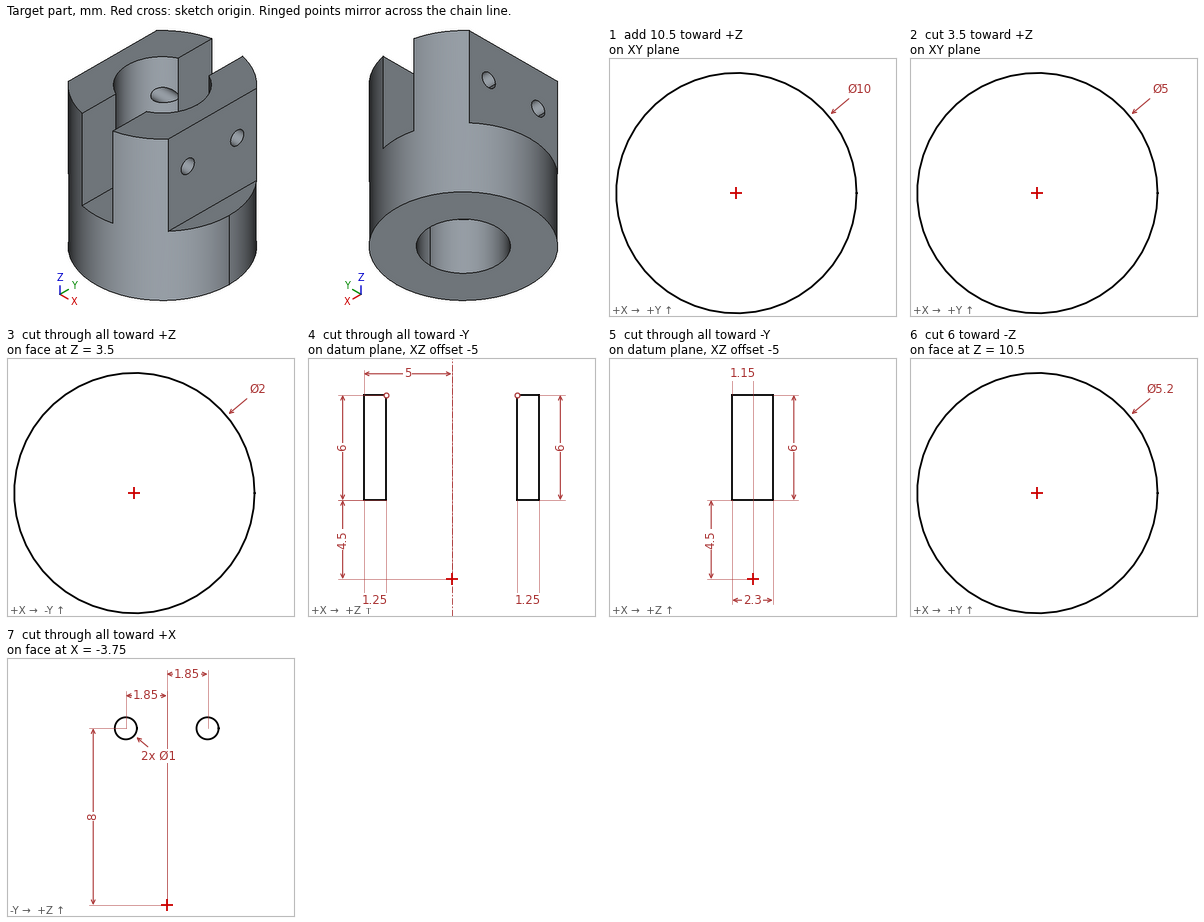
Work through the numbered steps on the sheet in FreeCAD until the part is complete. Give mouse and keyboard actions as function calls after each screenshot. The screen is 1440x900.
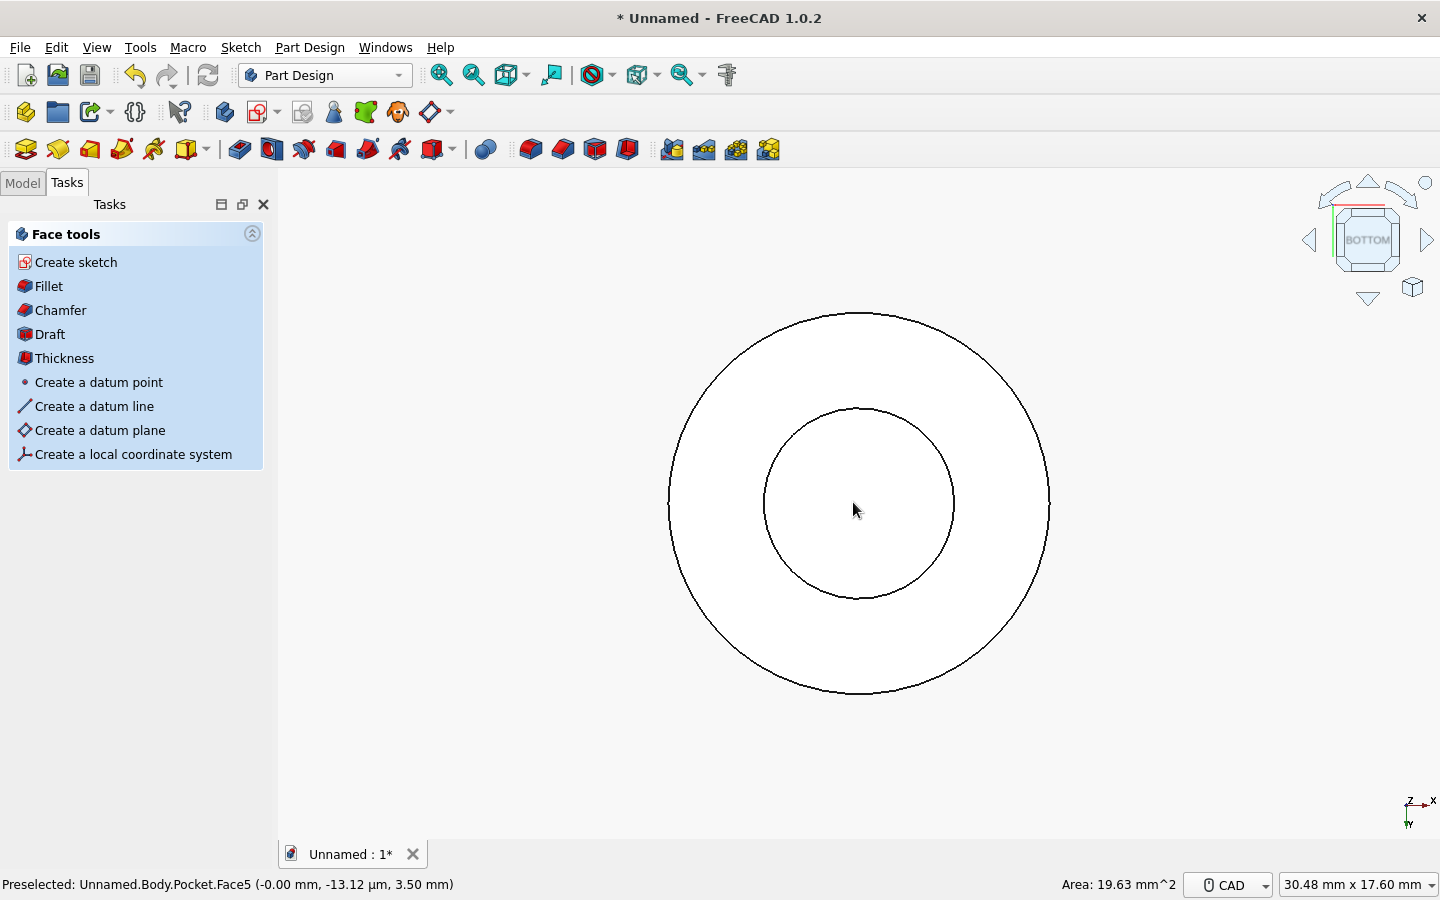
click(258, 112)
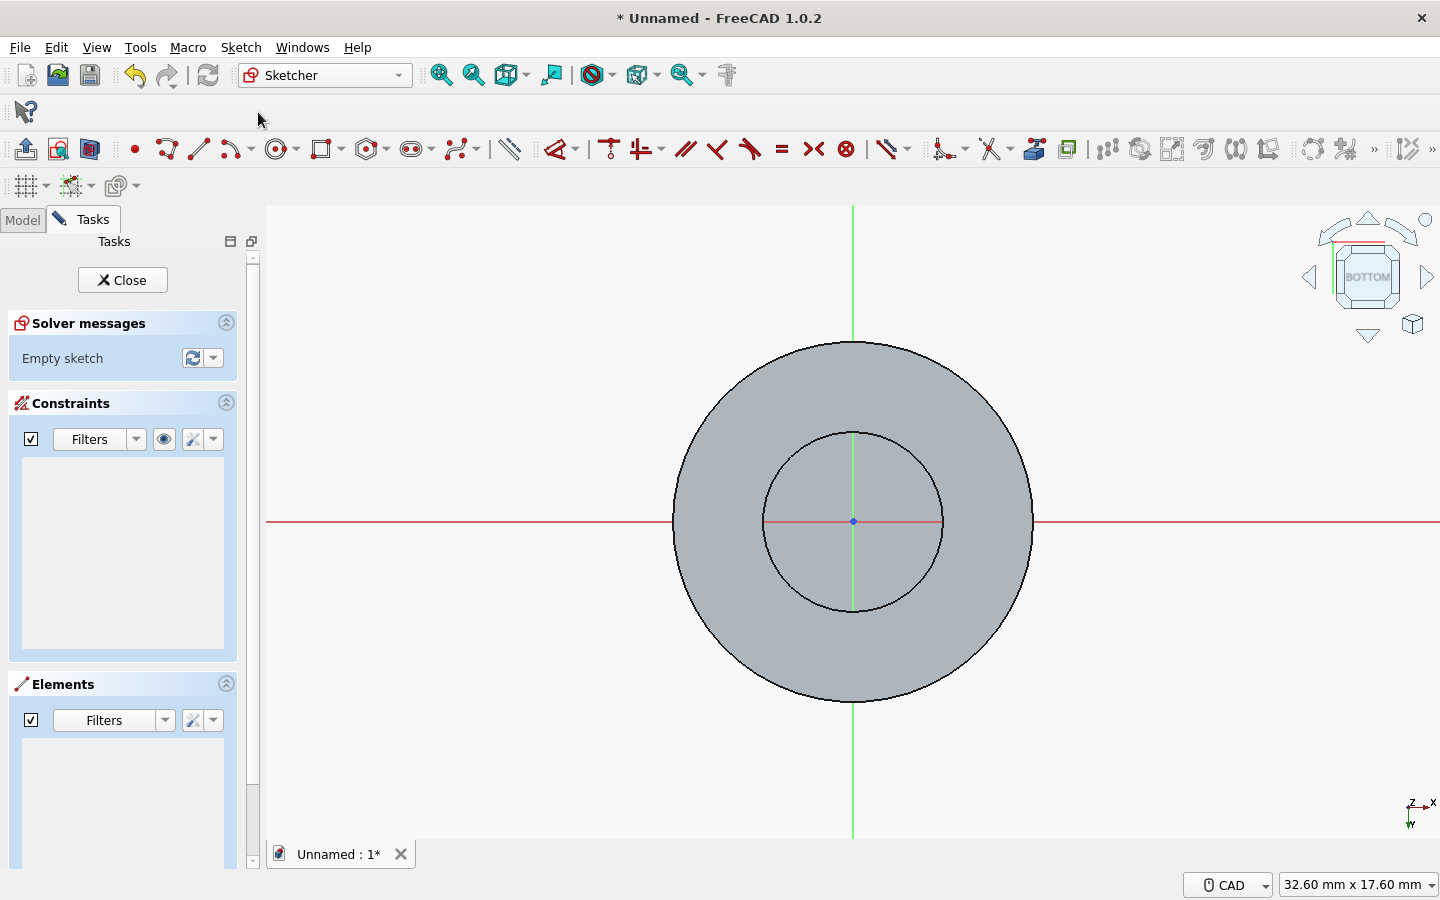
key(q)
key(s)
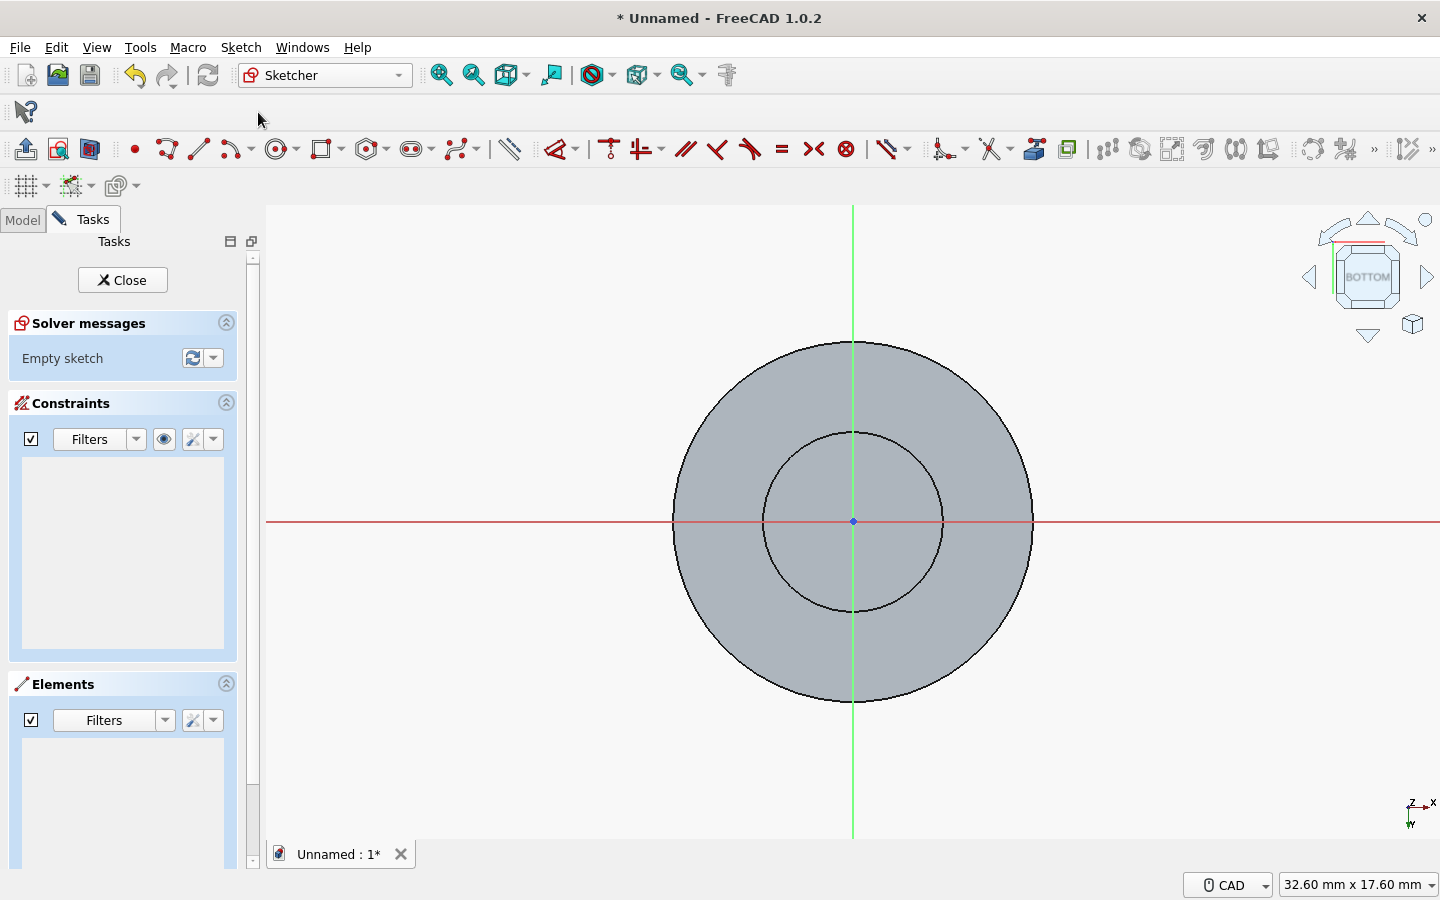
scroll(867, 522, up, 9)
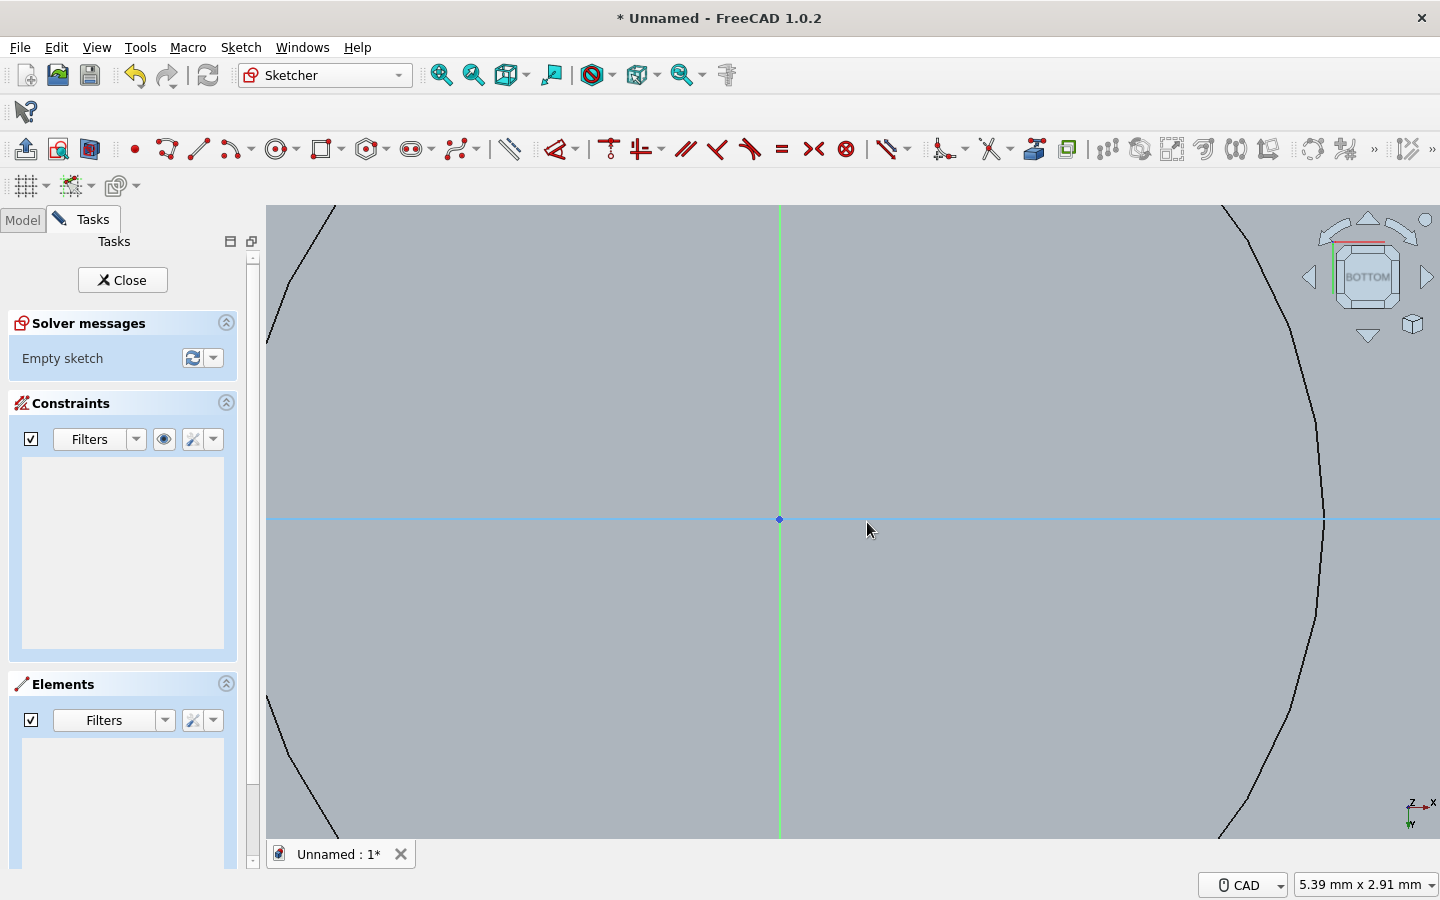
click(276, 150)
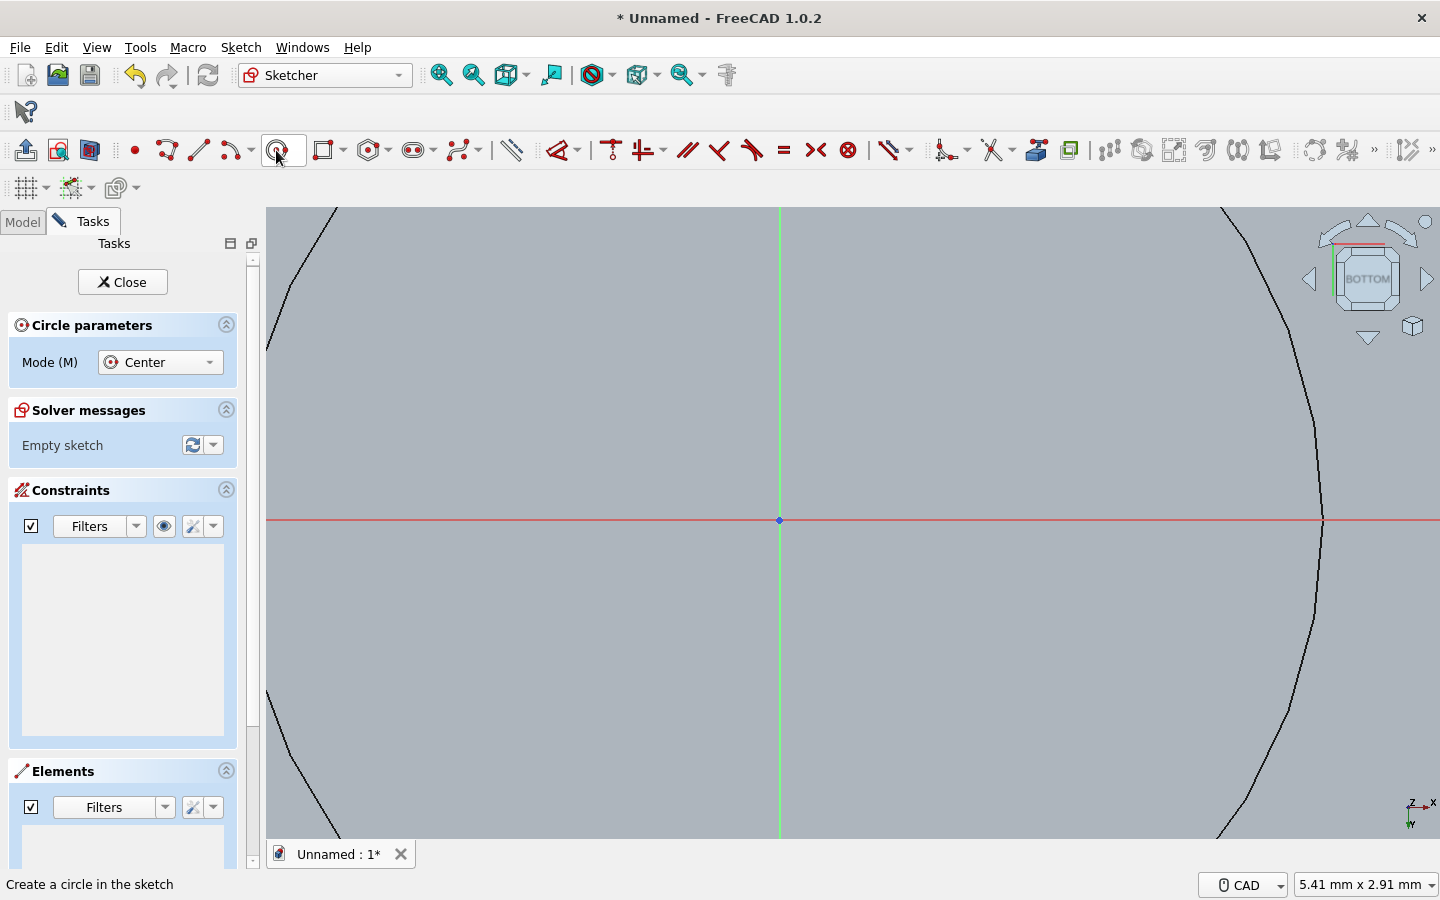
click(780, 520)
move(934, 367)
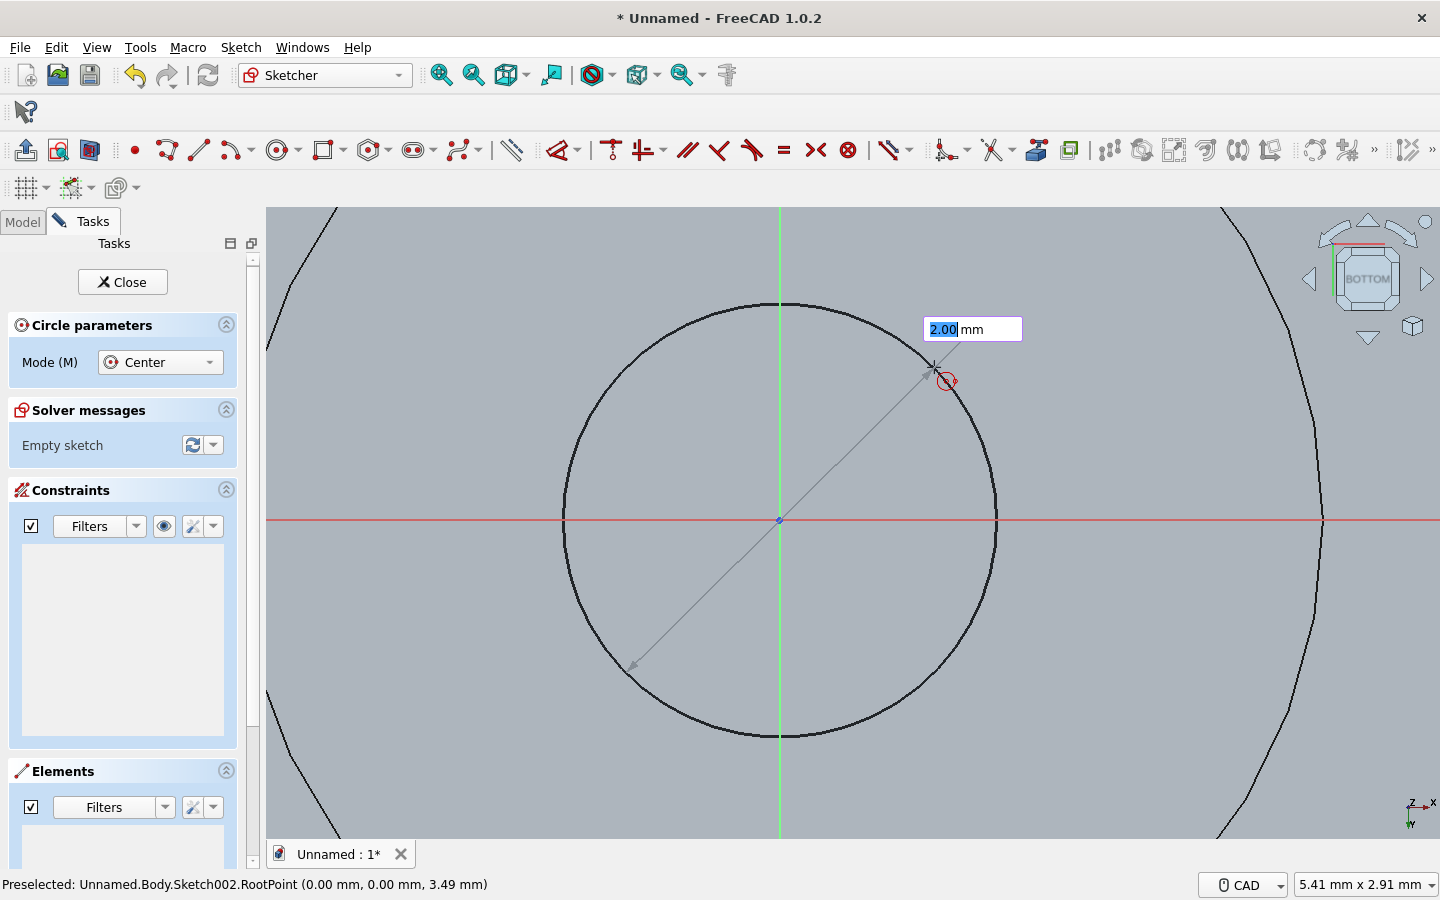
text(2)
key(Return)
key(Escape)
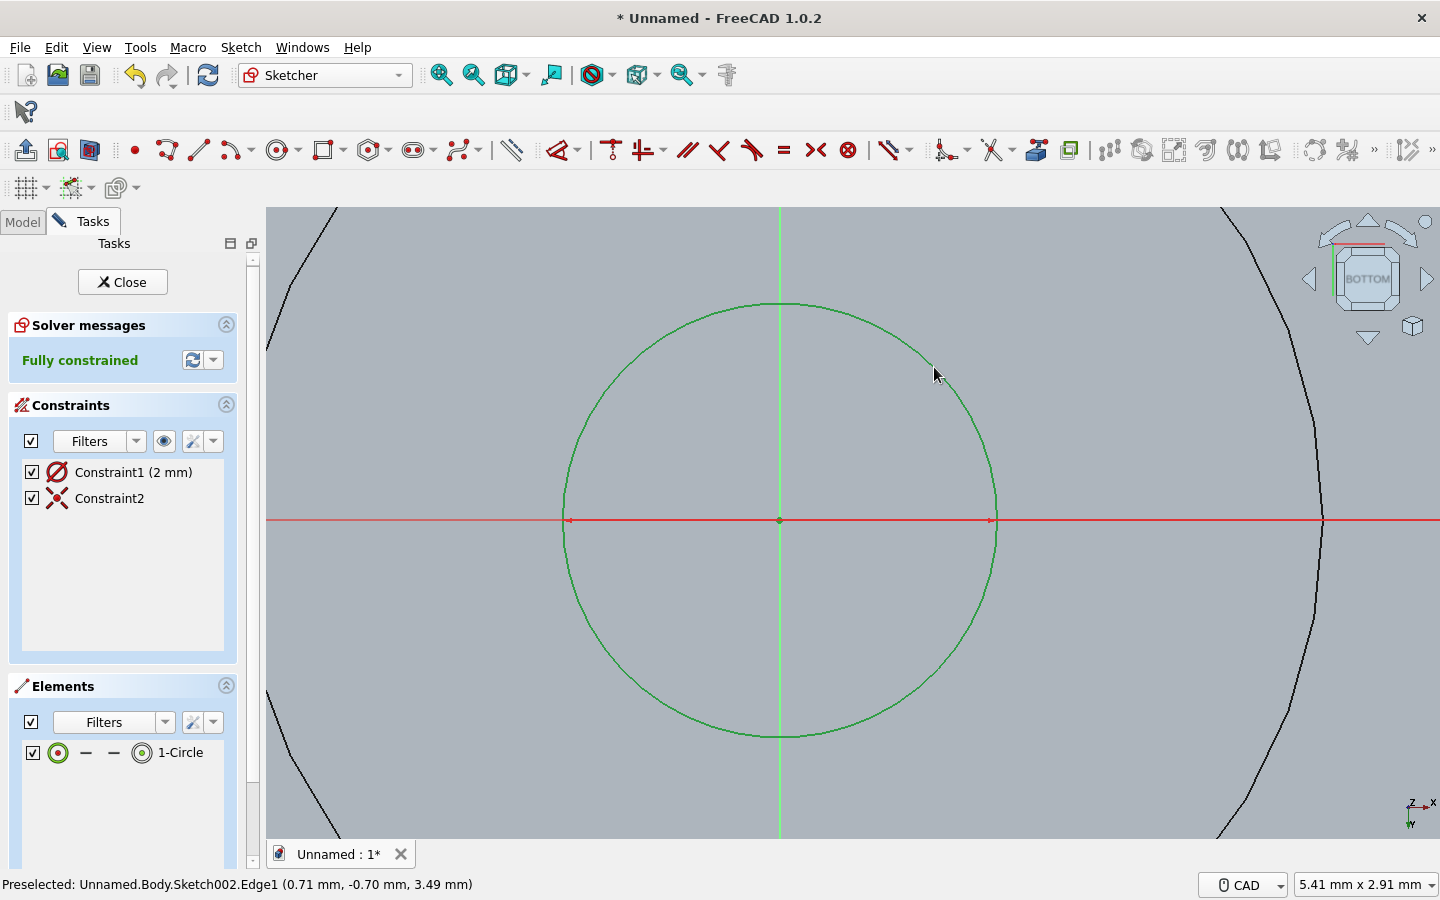
click(123, 282)